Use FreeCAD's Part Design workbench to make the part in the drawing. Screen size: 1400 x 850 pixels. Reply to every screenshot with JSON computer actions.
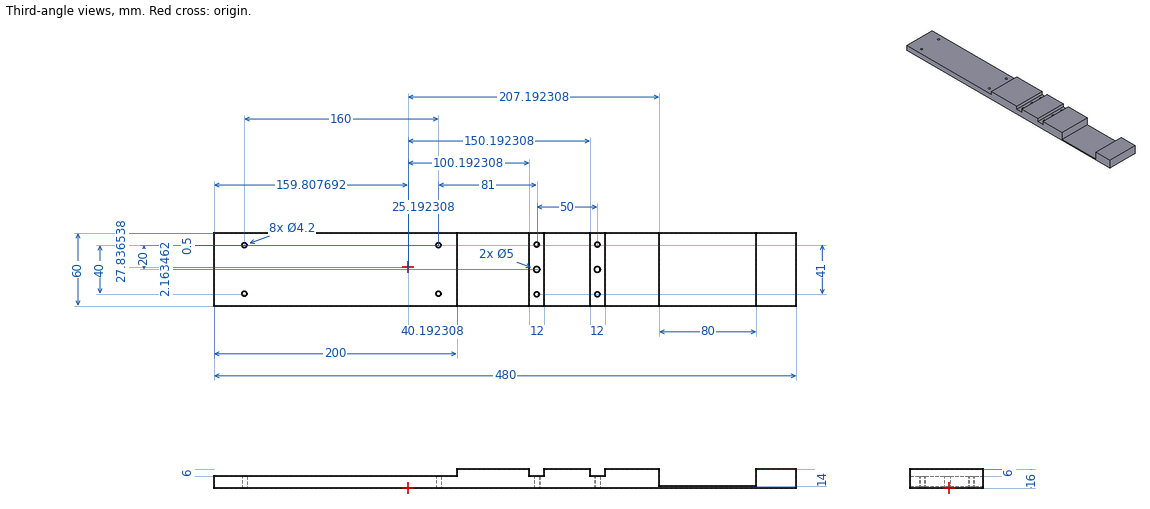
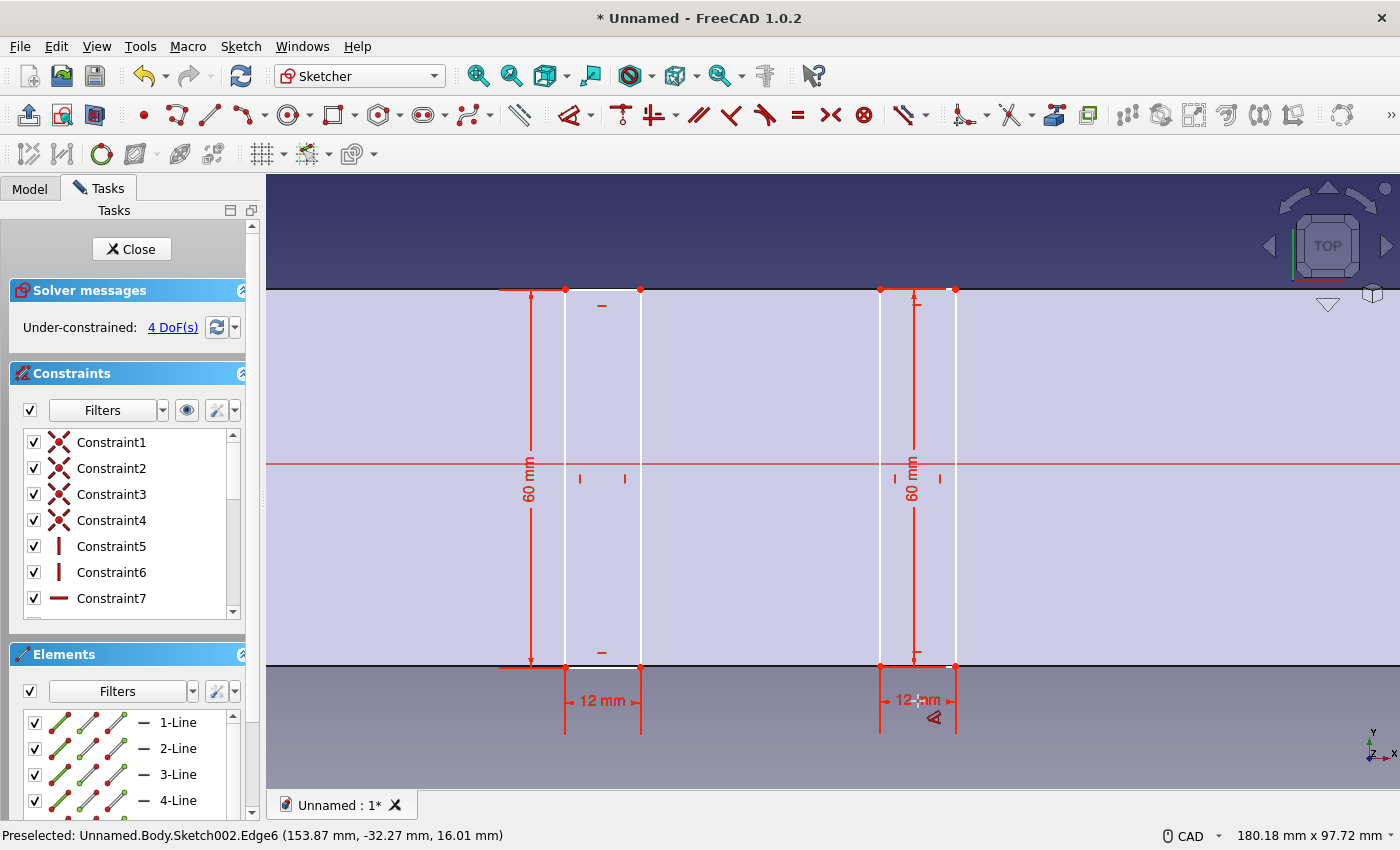
{"action": "left_click", "coordinate": [565, 290]}
{"action": "left_click", "coordinate": [599, 377]}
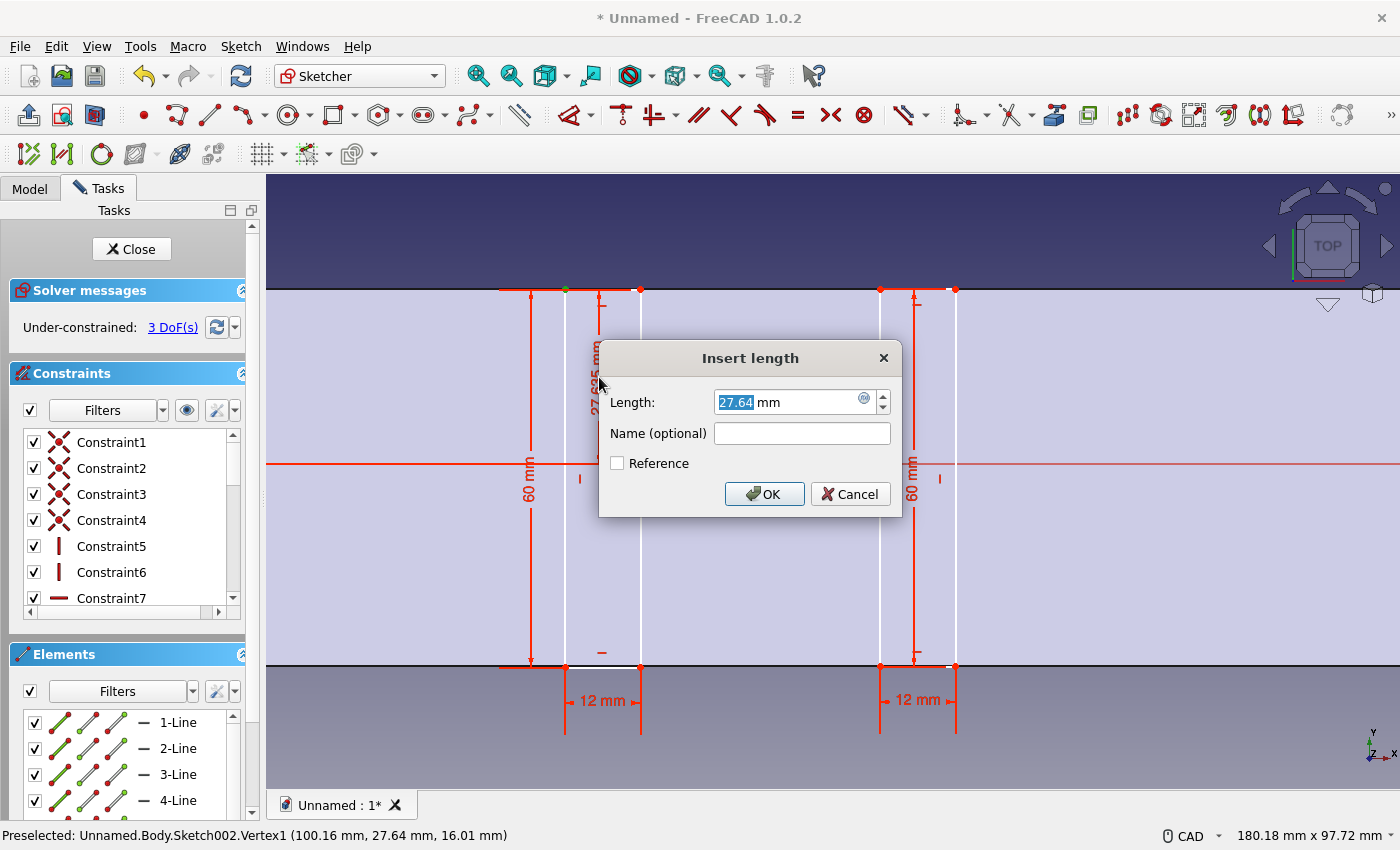
{"action": "type", "text": "27.836538"}
{"action": "key", "text": "Return"}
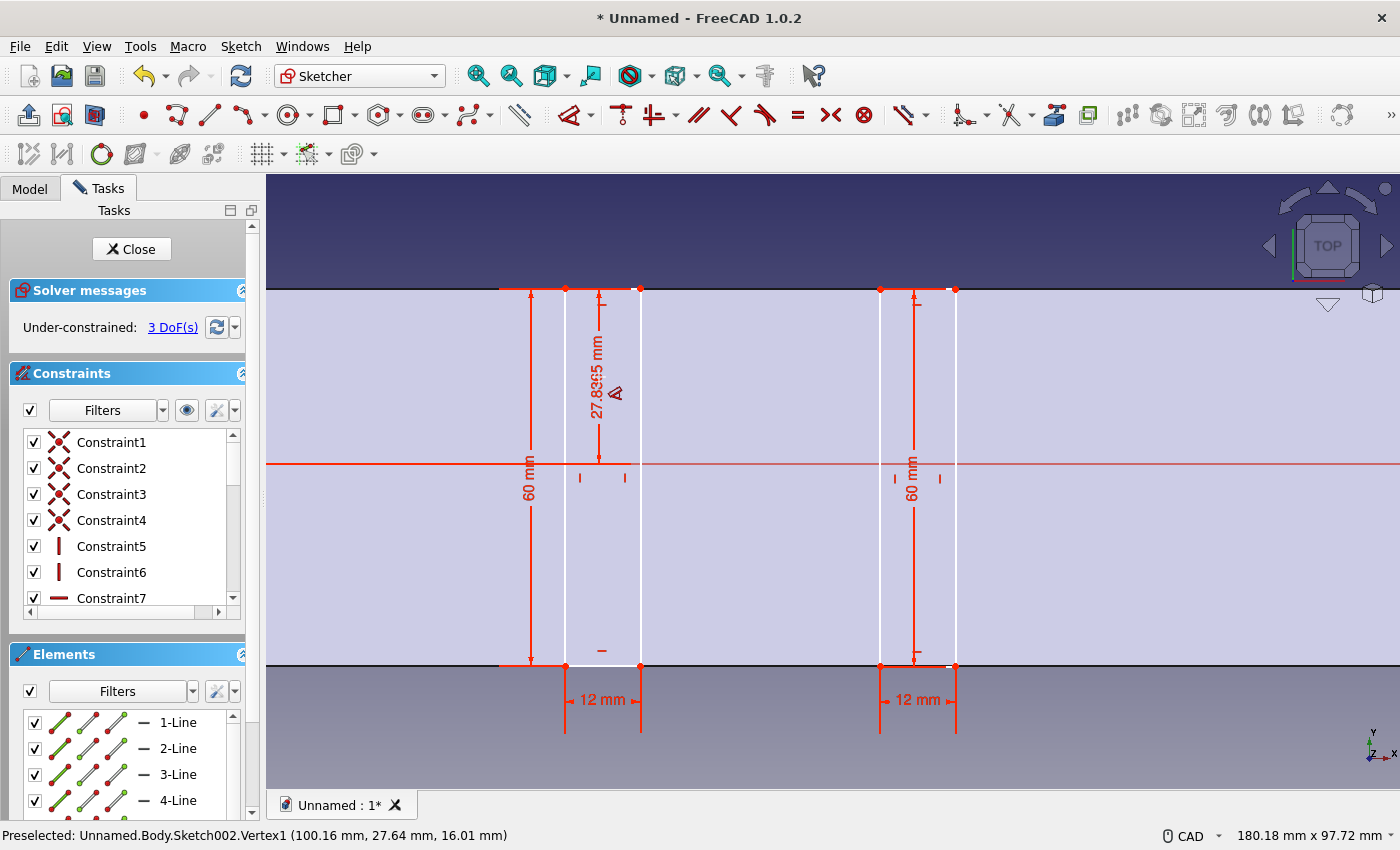
{"action": "left_click", "coordinate": [880, 289]}
{"action": "left_click", "coordinate": [914, 377]}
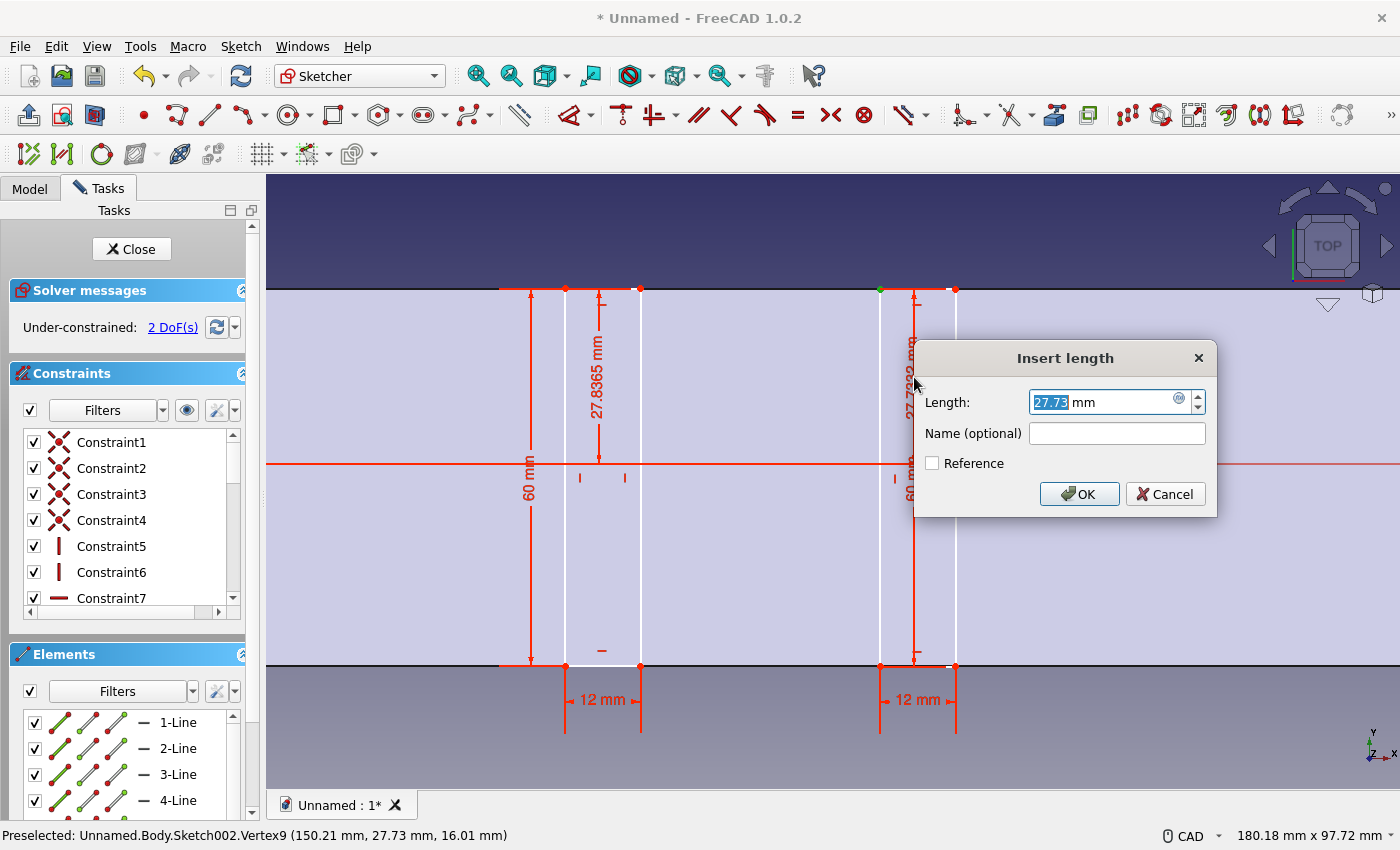
{"action": "type", "text": "27.836538"}
{"action": "key", "text": "Return"}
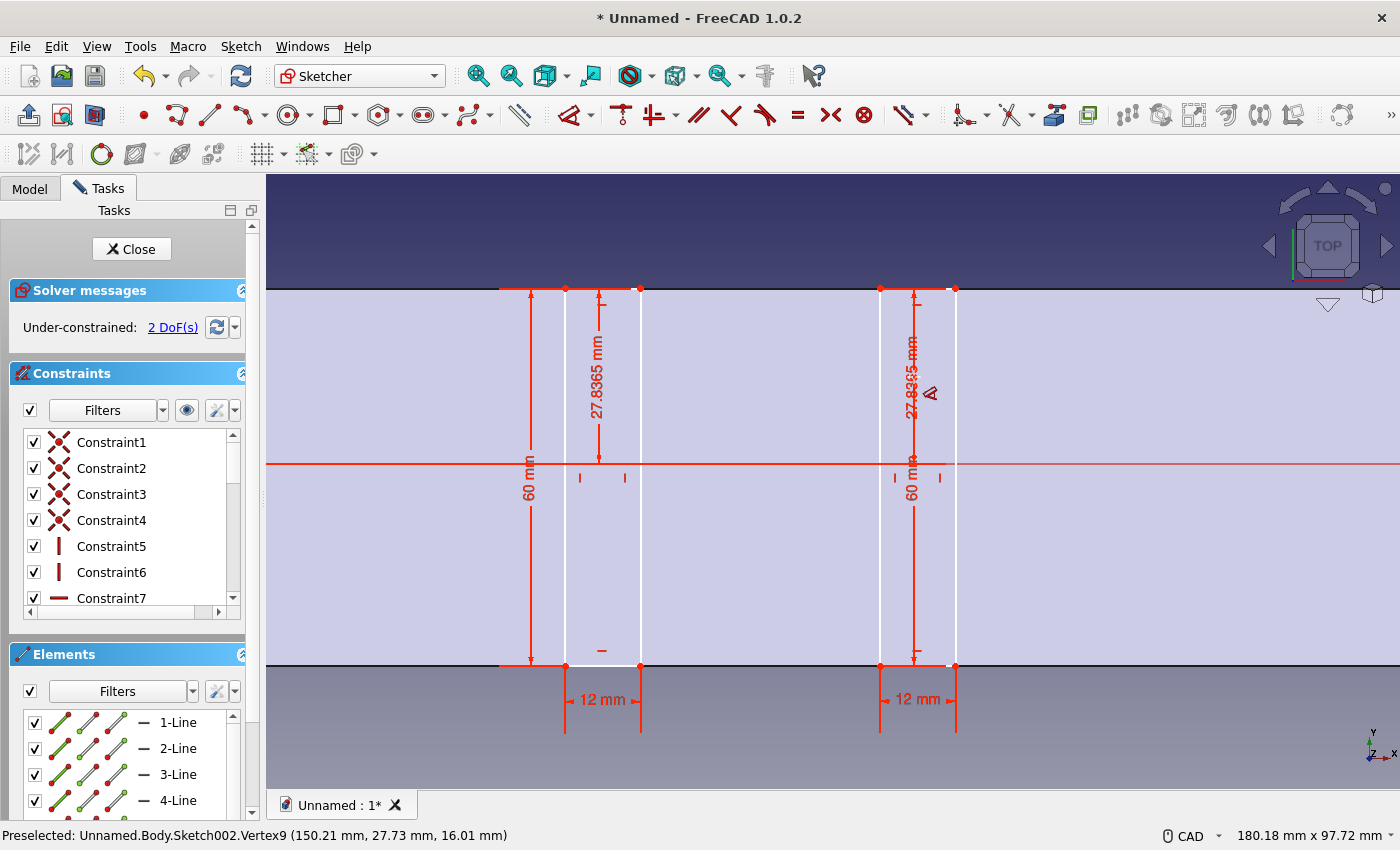
{"action": "left_click", "coordinate": [565, 289]}
{"action": "left_click", "coordinate": [430, 255]}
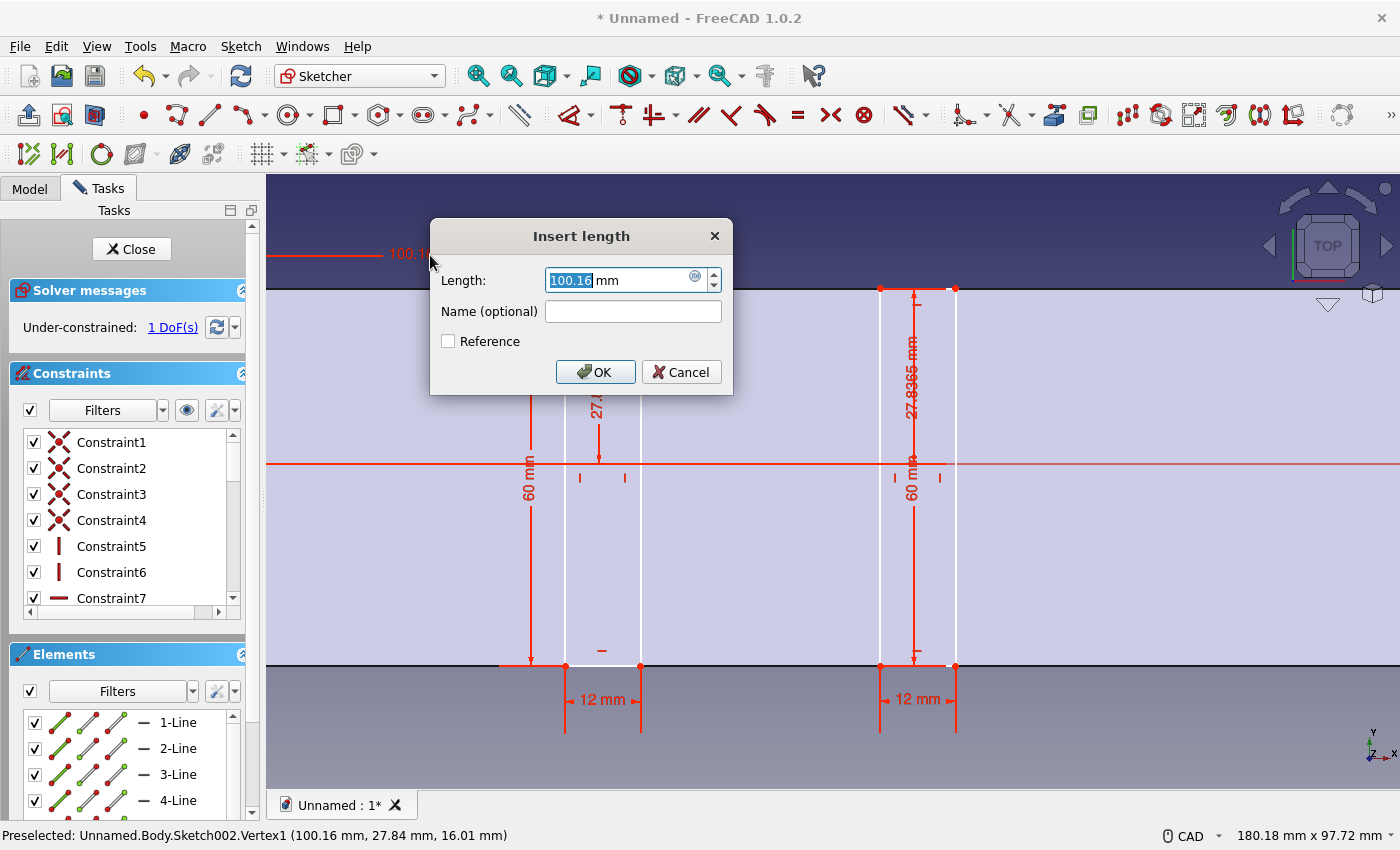
{"action": "type", "text": "100.192308"}
{"action": "key", "text": "Return"}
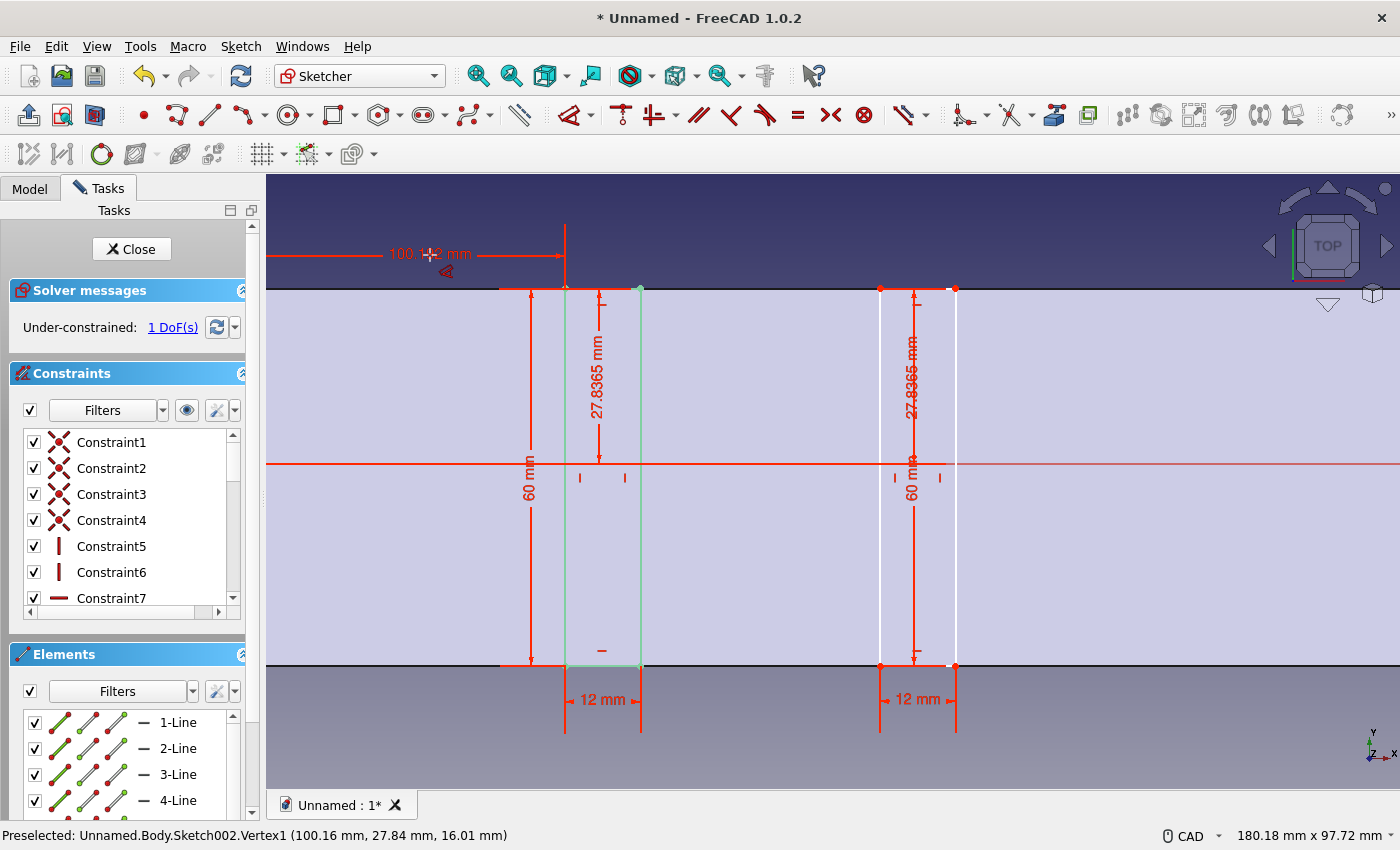
{"action": "left_click", "coordinate": [880, 289]}
{"action": "left_click", "coordinate": [587, 255]}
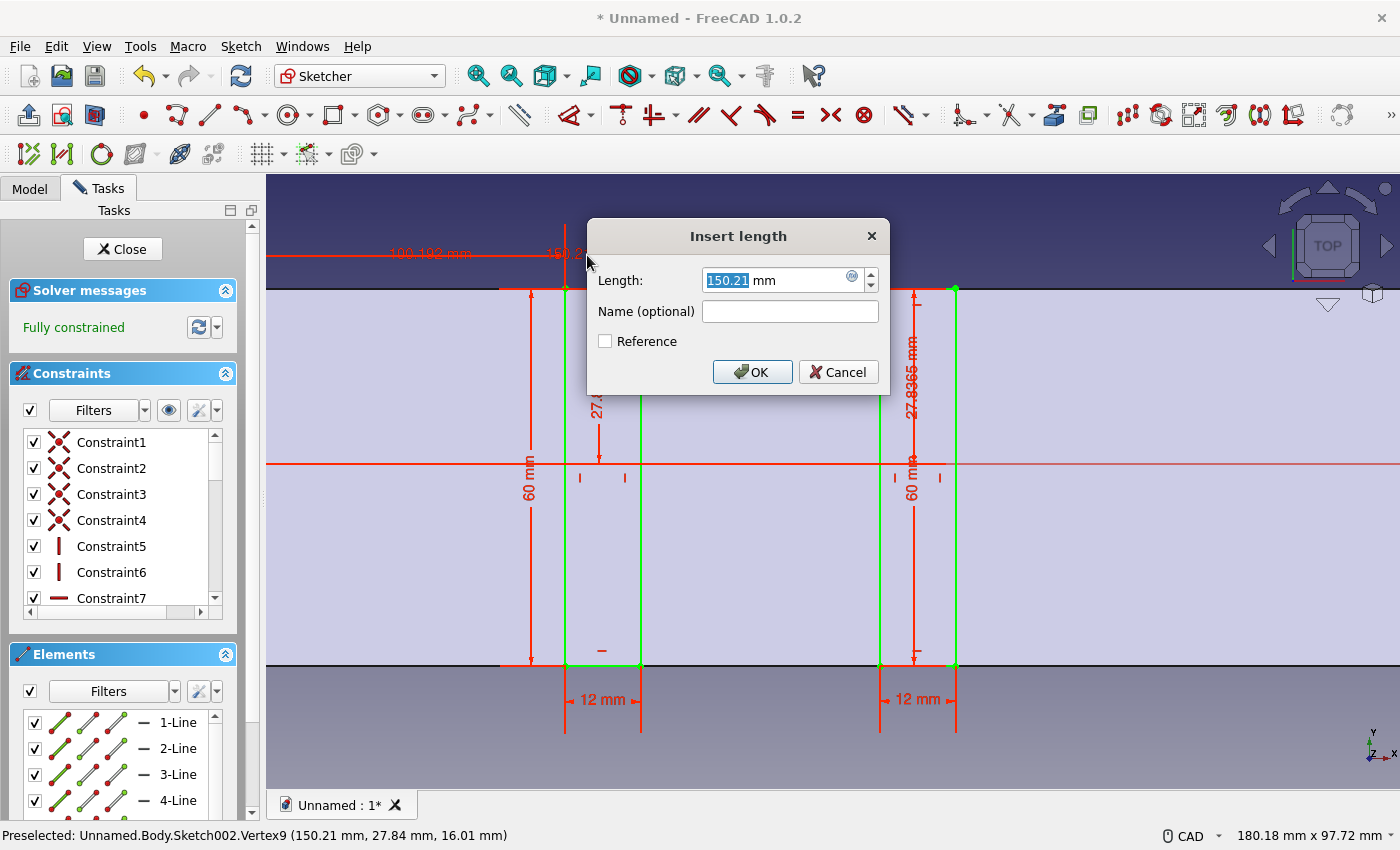
{"action": "type", "text": "150.192308"}
{"action": "key", "text": "Return"}
{"action": "key", "text": "Escape"}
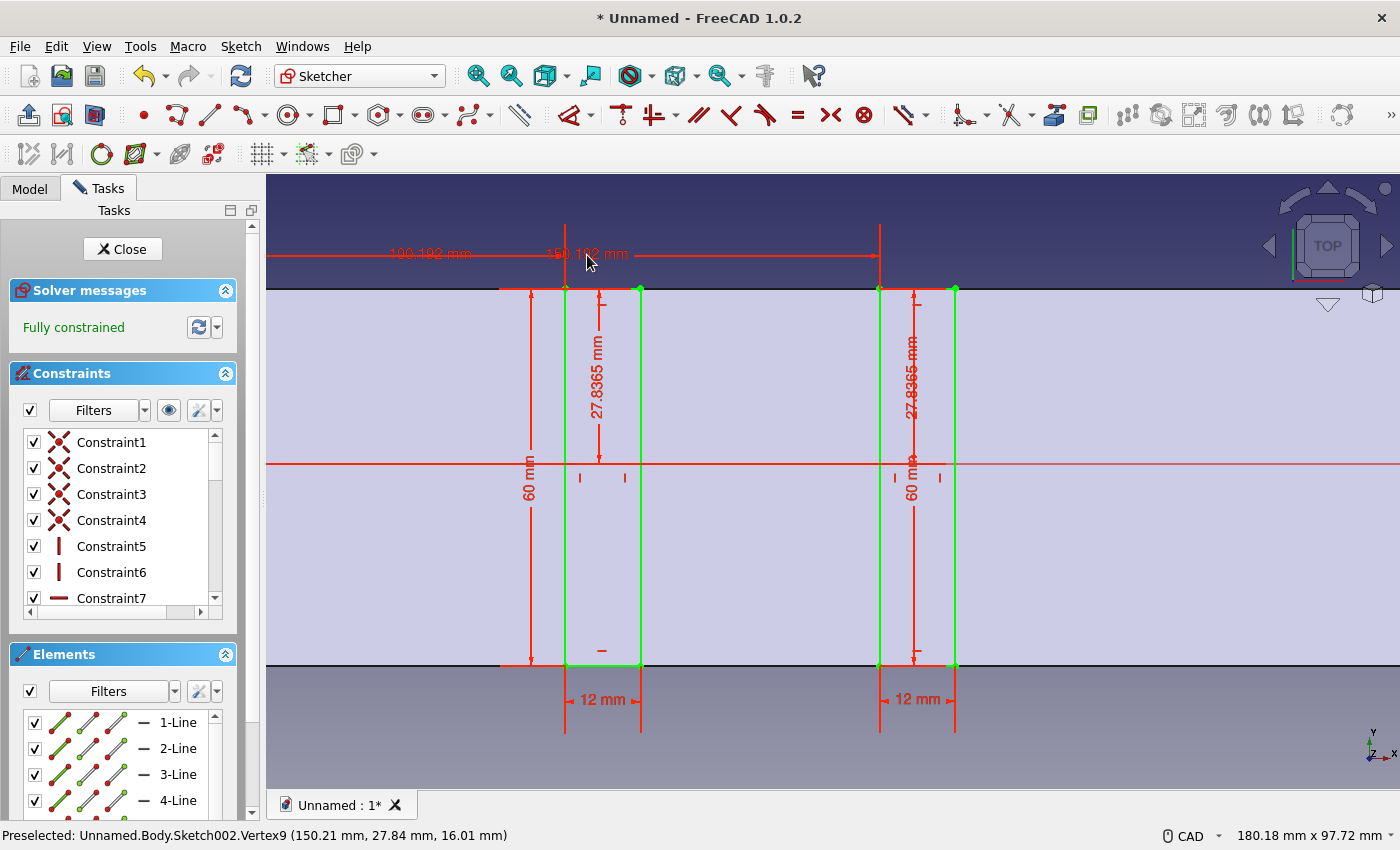
{"action": "left_click", "coordinate": [123, 249]}